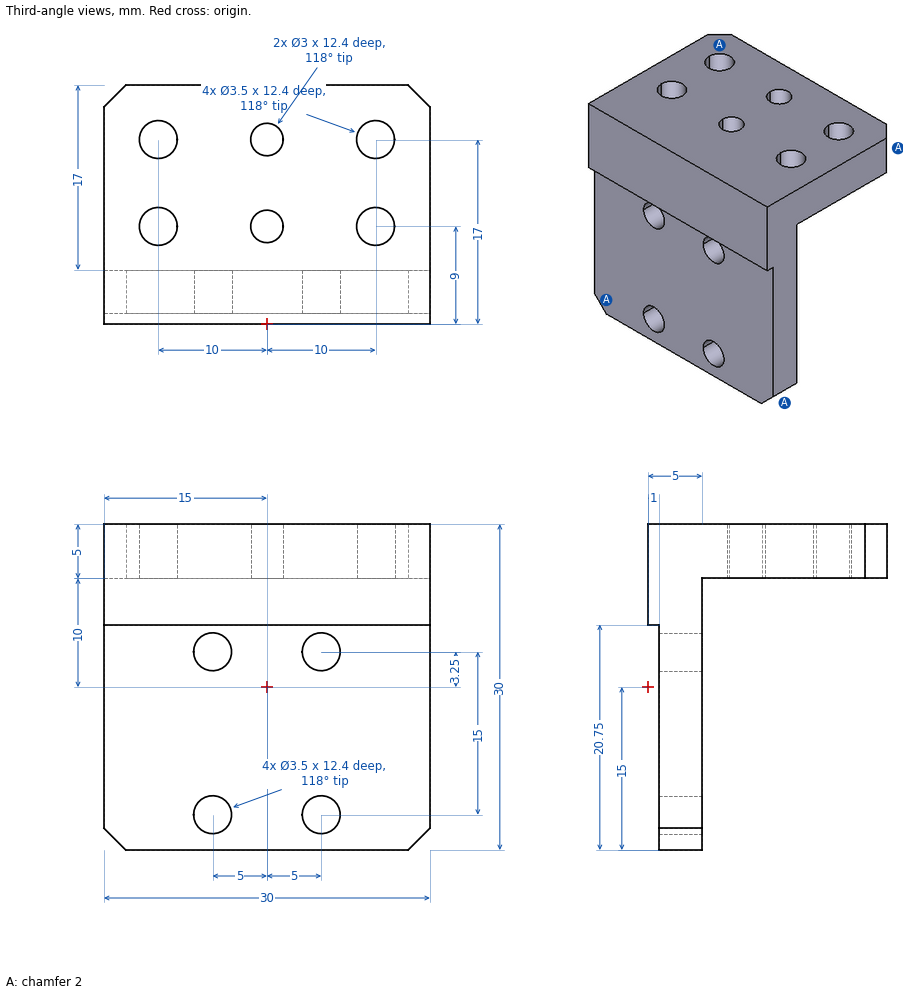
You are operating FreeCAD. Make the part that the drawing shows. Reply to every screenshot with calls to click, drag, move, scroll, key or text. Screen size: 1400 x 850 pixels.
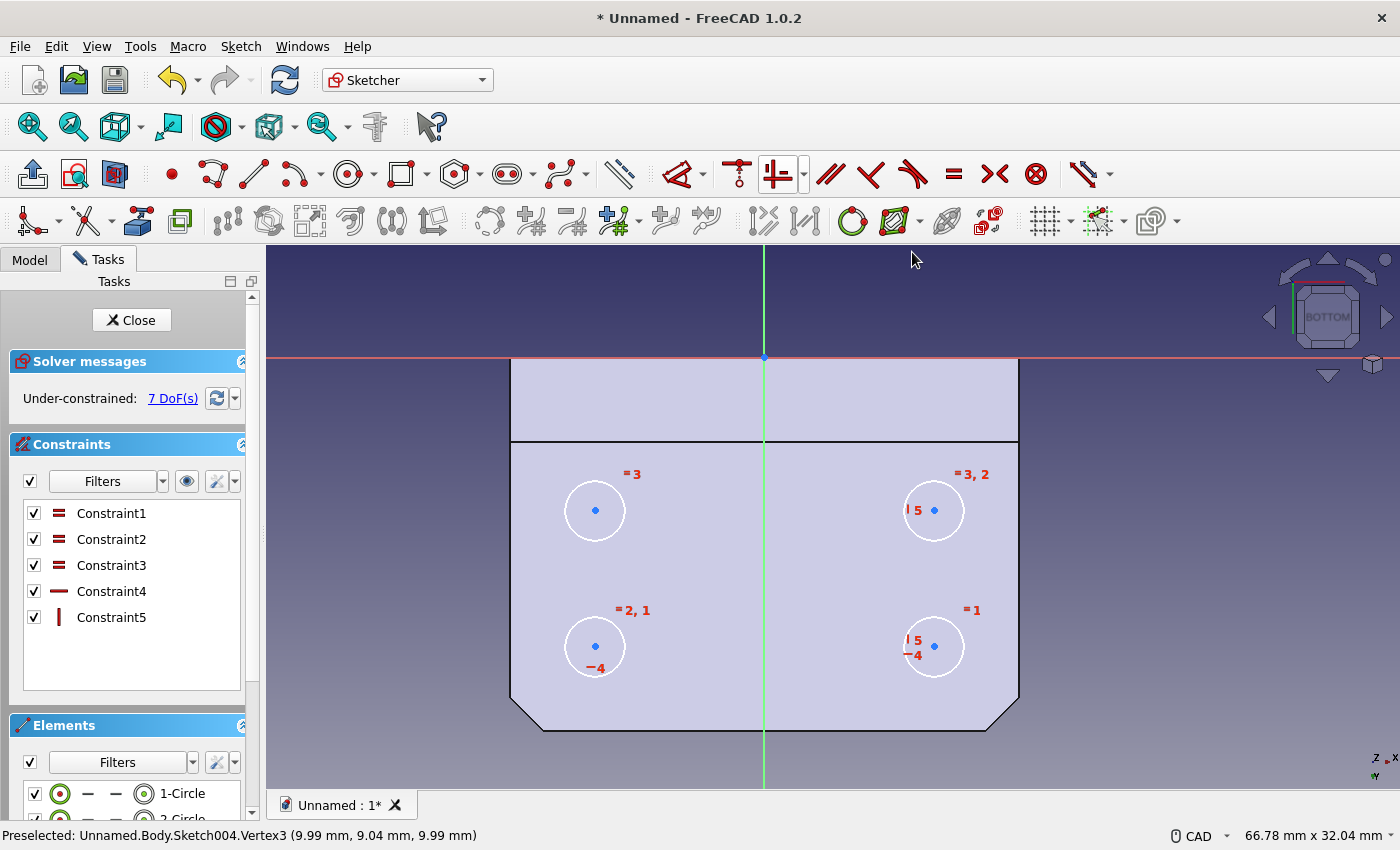
click(595, 647)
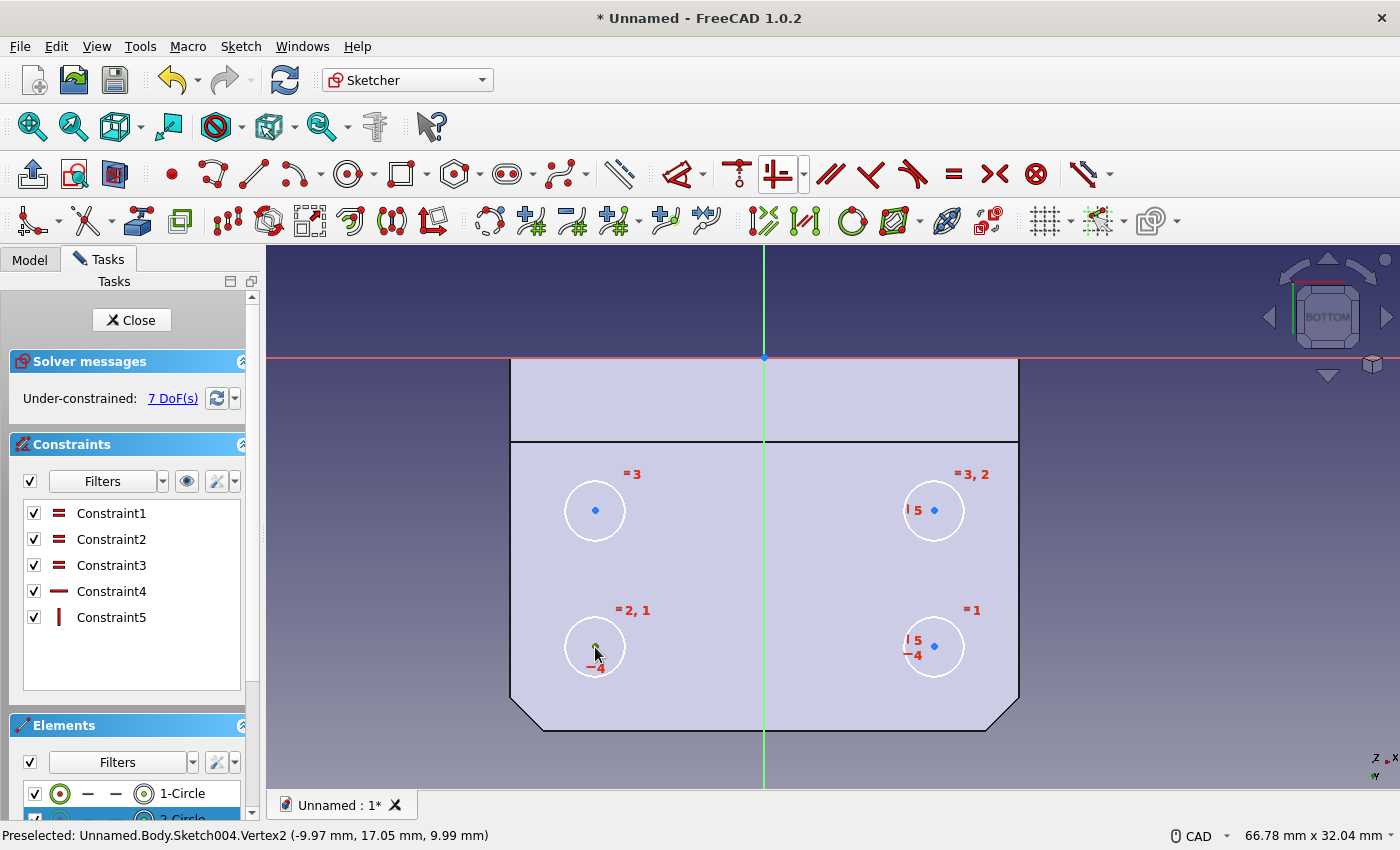
click(595, 511)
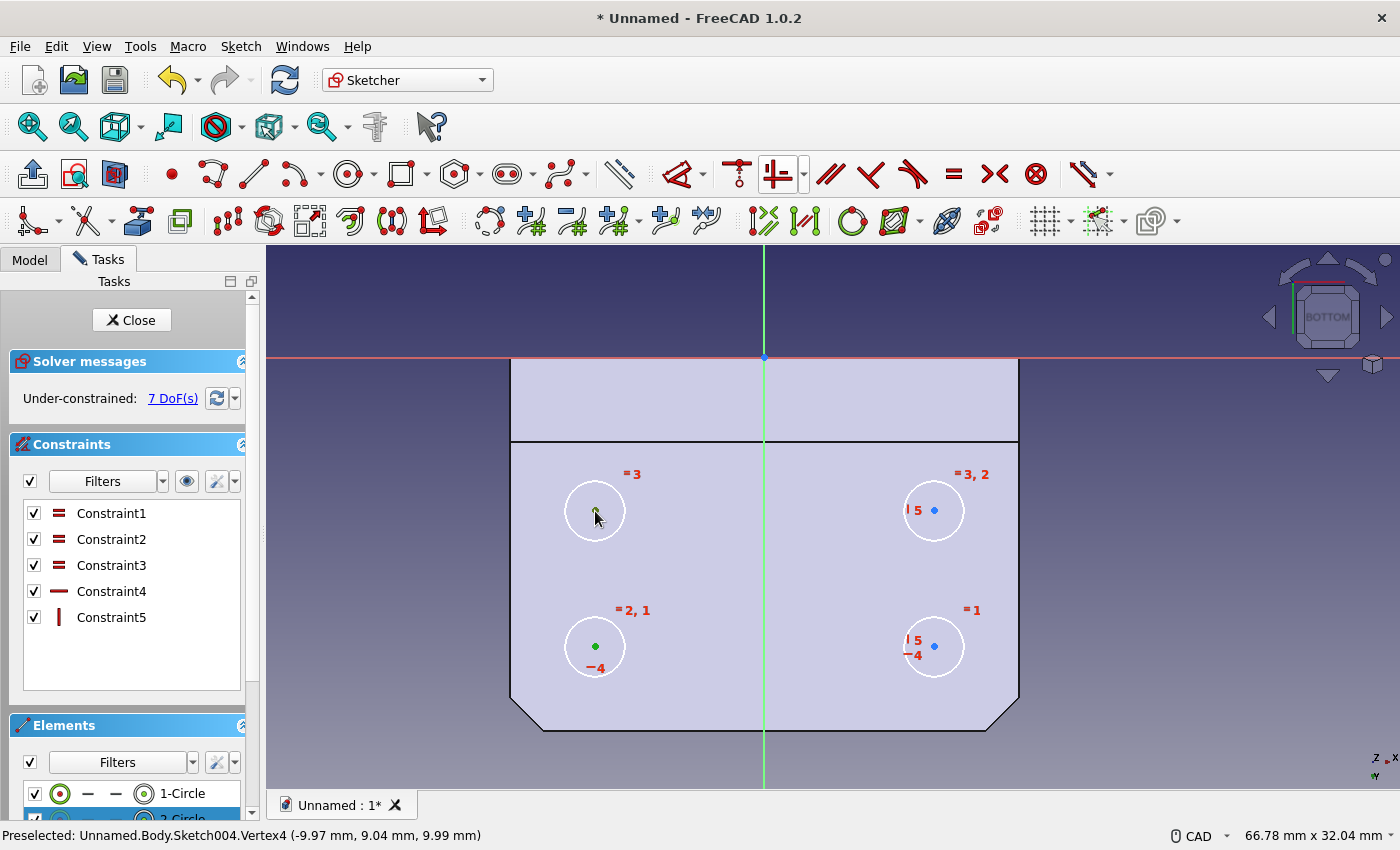
key(v)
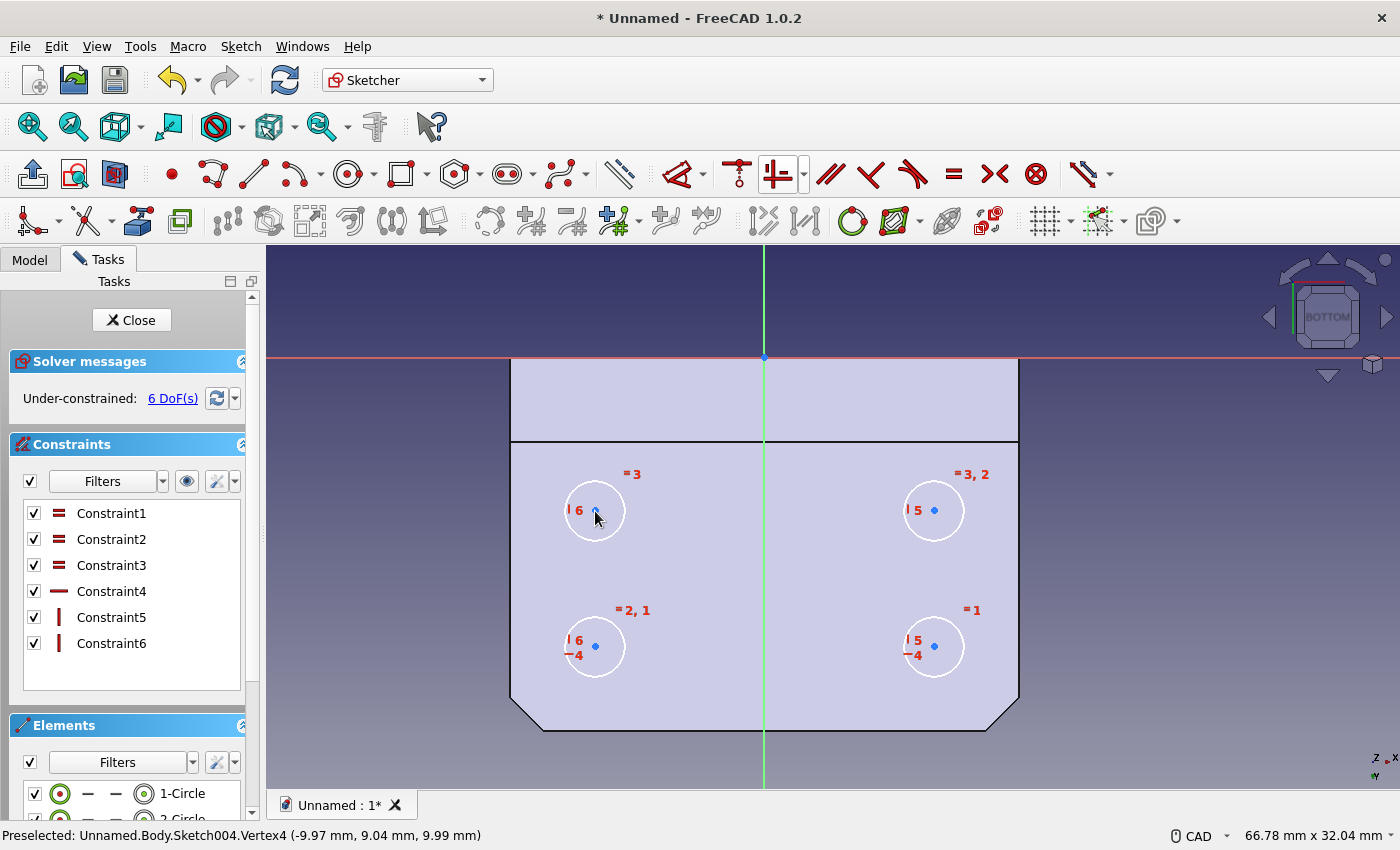
click(934, 511)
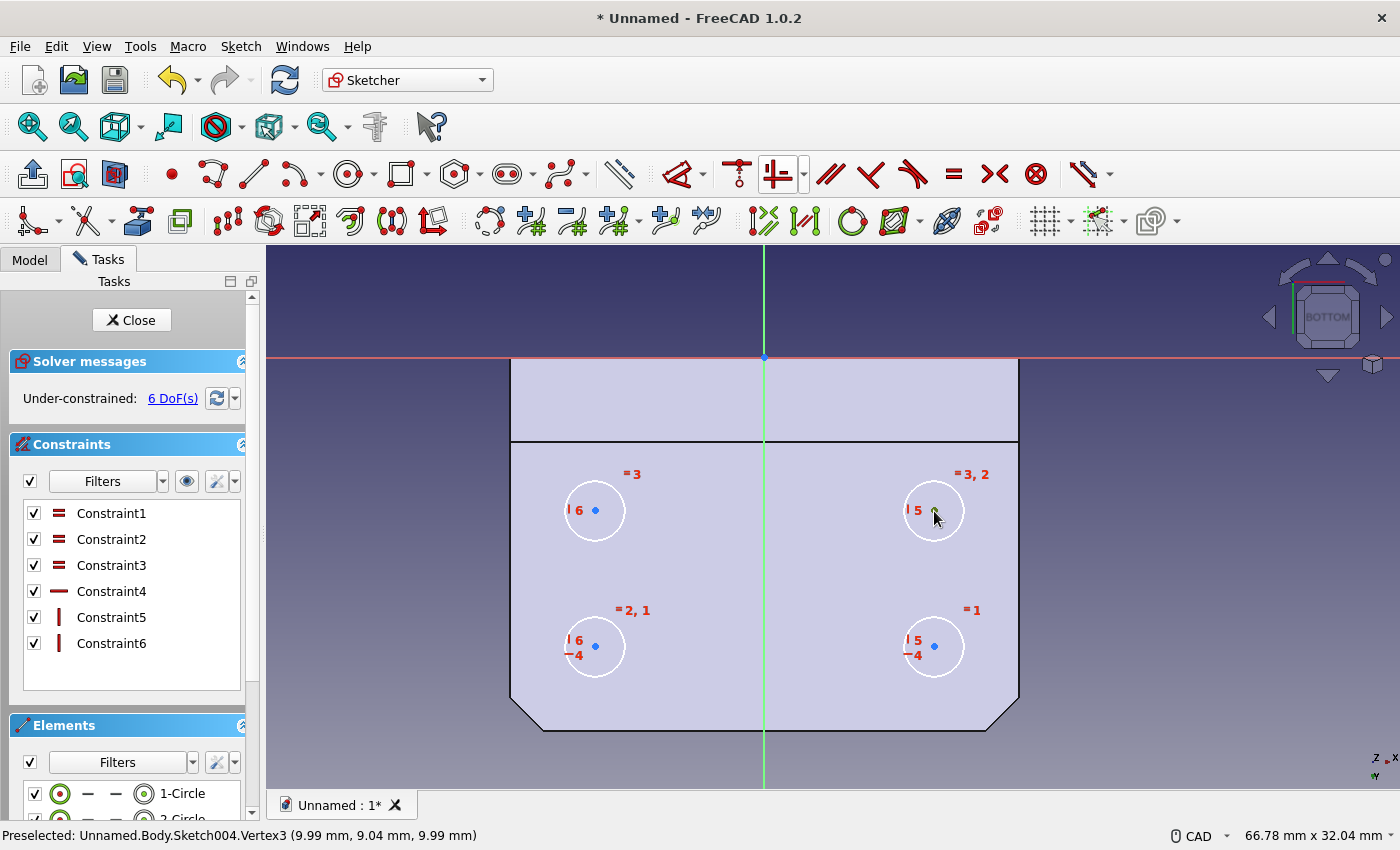
click(595, 511)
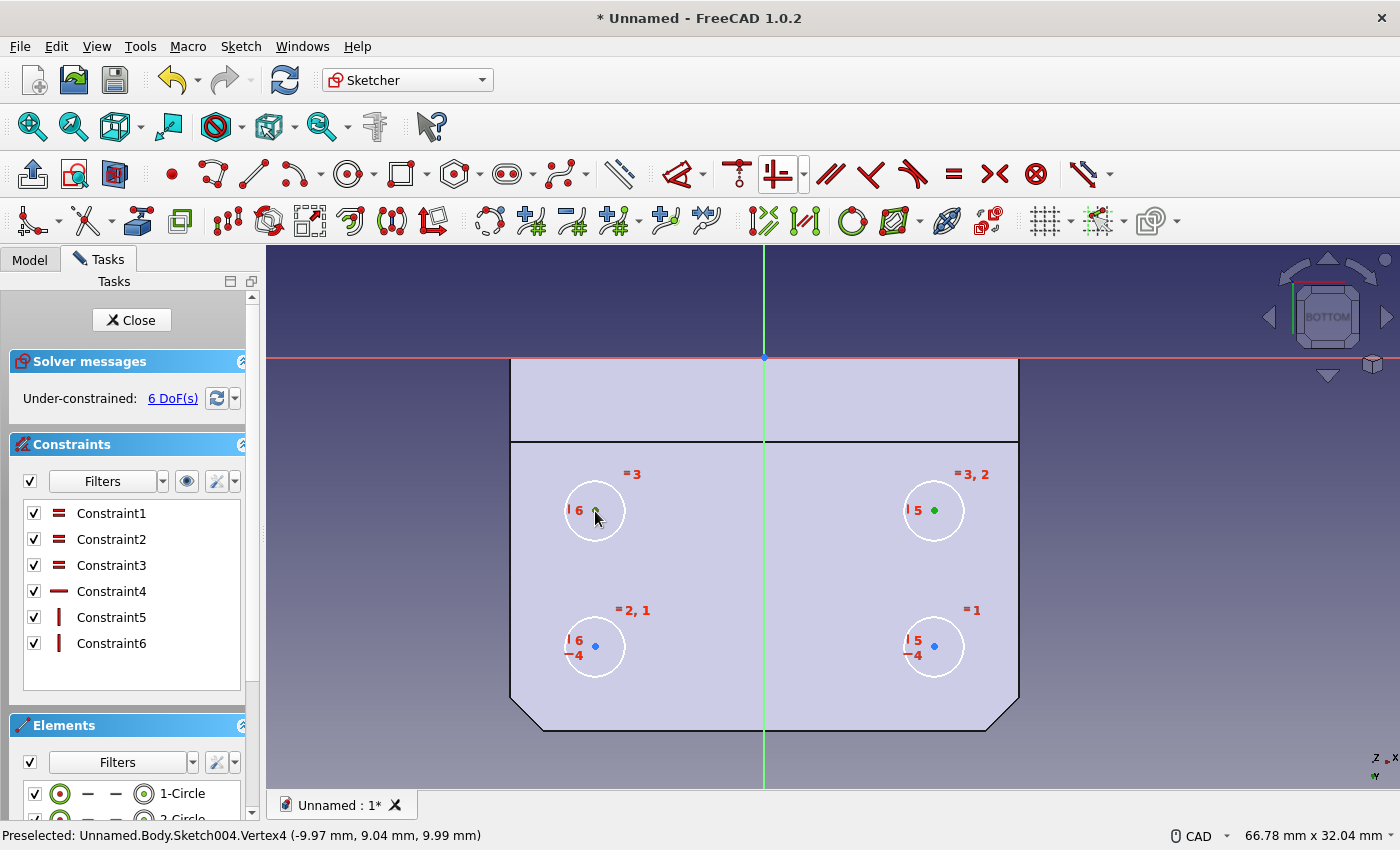
key(h)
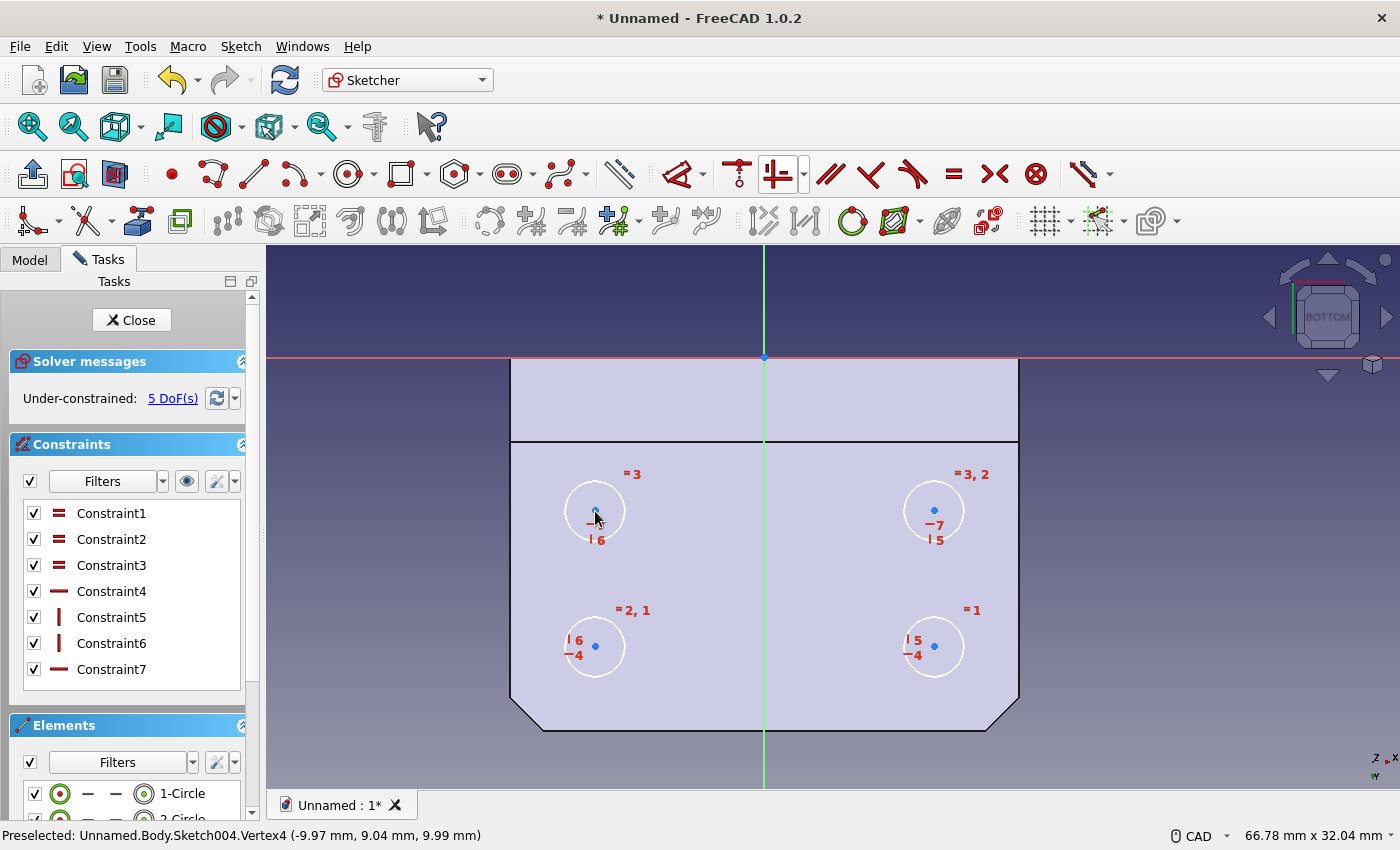
key(d)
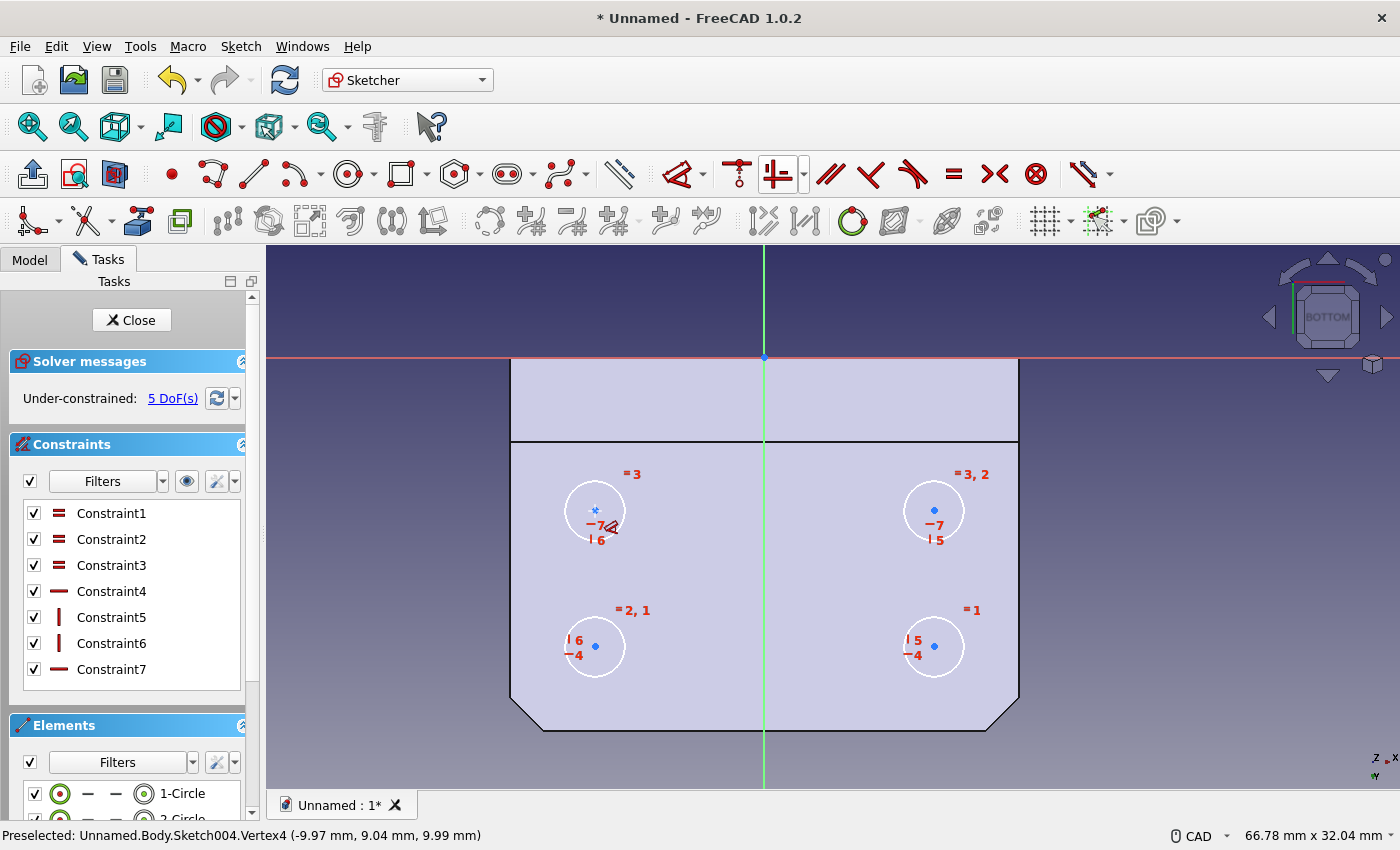
click(955, 626)
click(978, 603)